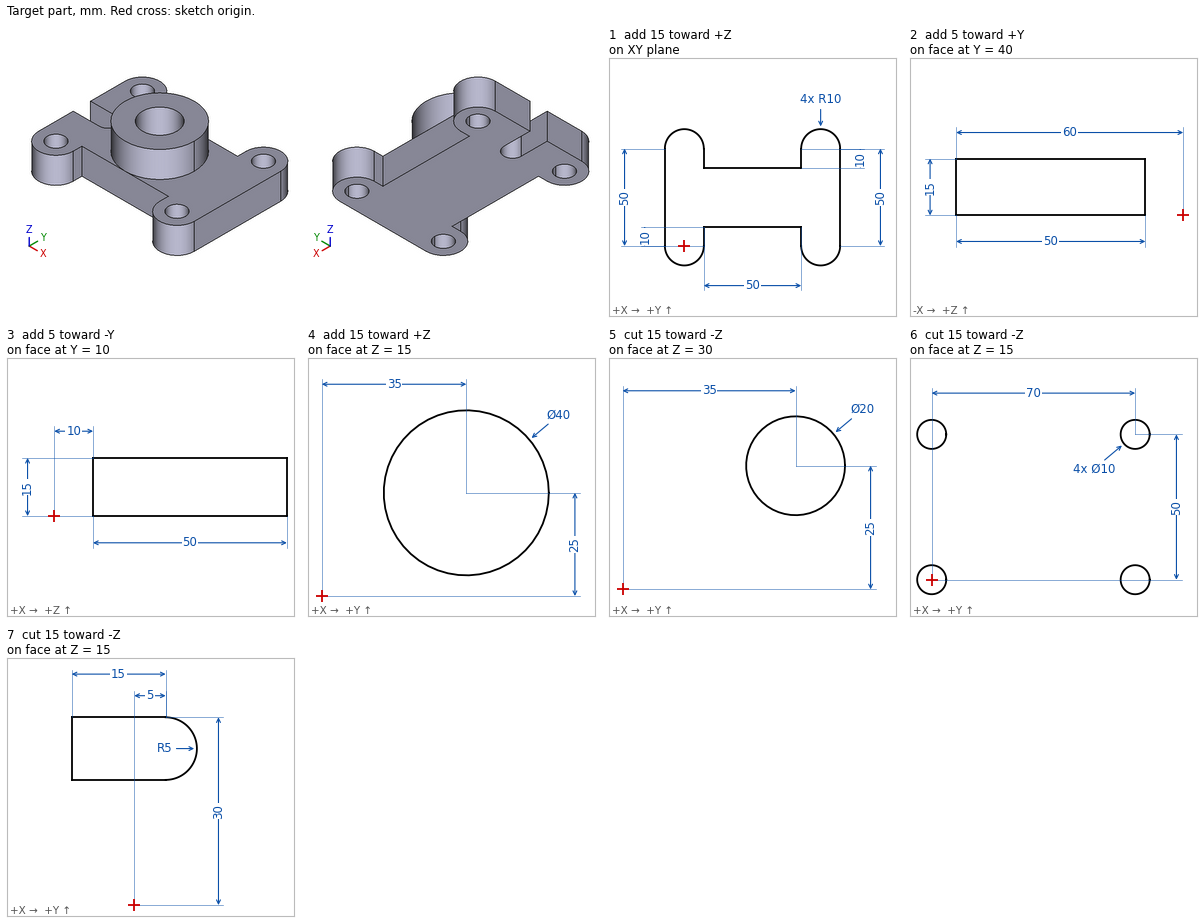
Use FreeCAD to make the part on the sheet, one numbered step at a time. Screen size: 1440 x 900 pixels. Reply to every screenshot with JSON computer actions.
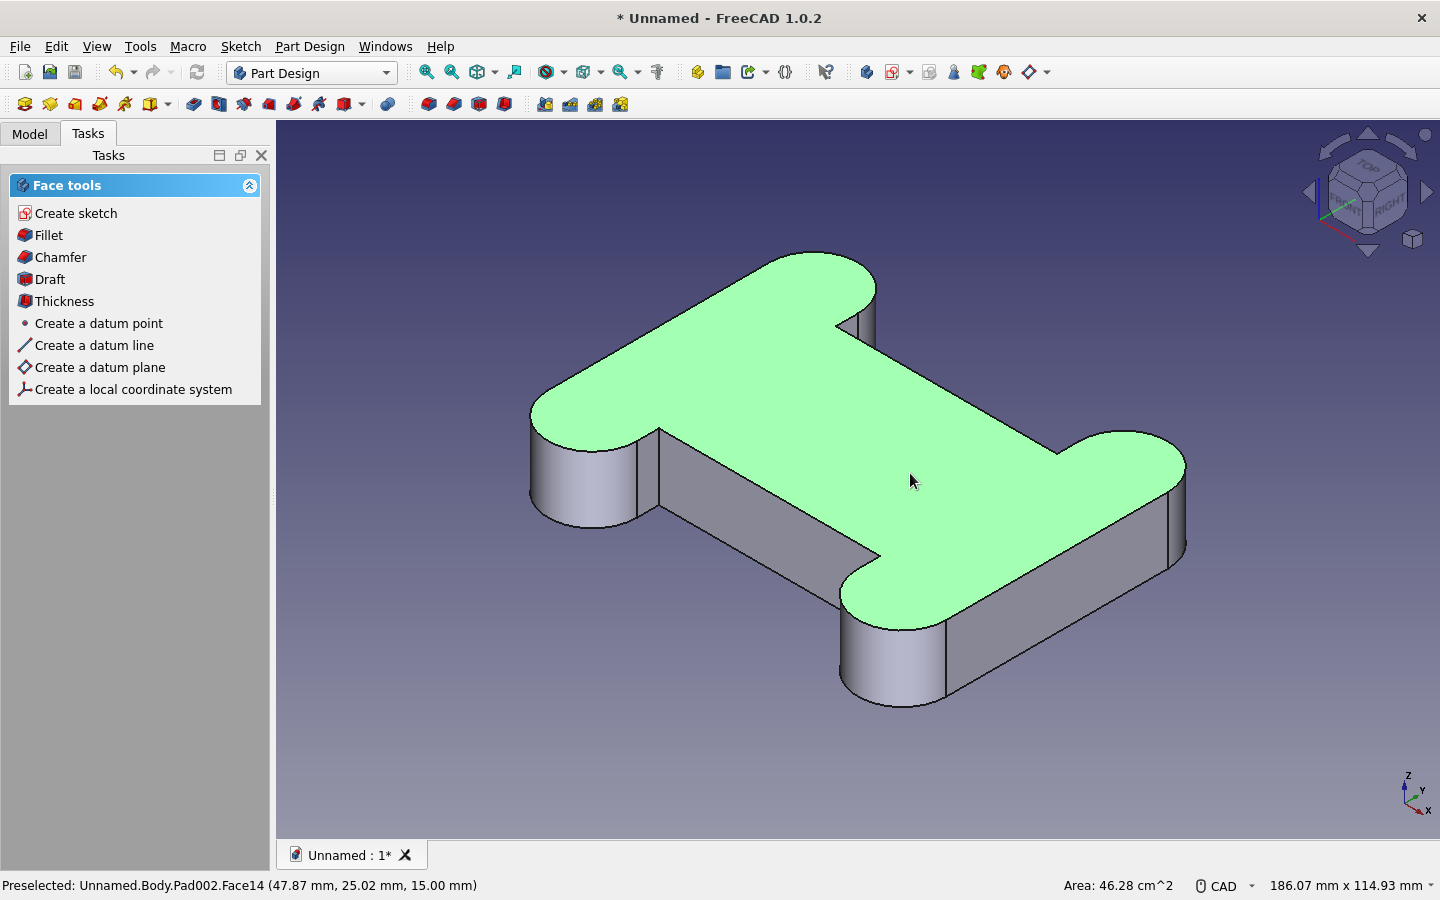
{"action": "left_click", "coordinate": [892, 72]}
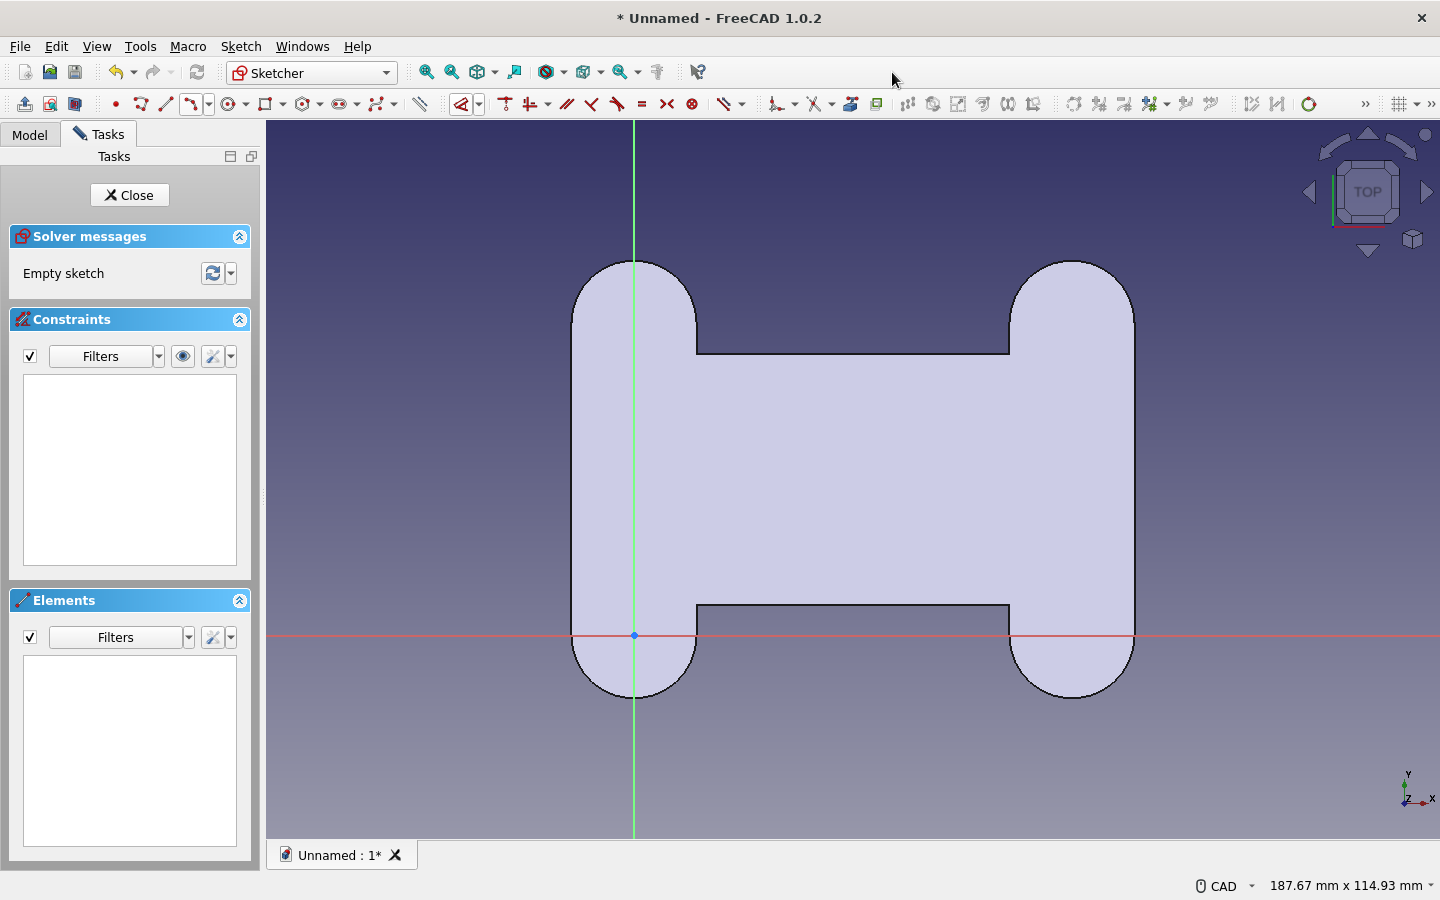
{"action": "scroll", "coordinate": [832, 514], "scroll_direction": "up", "scroll_amount": 3}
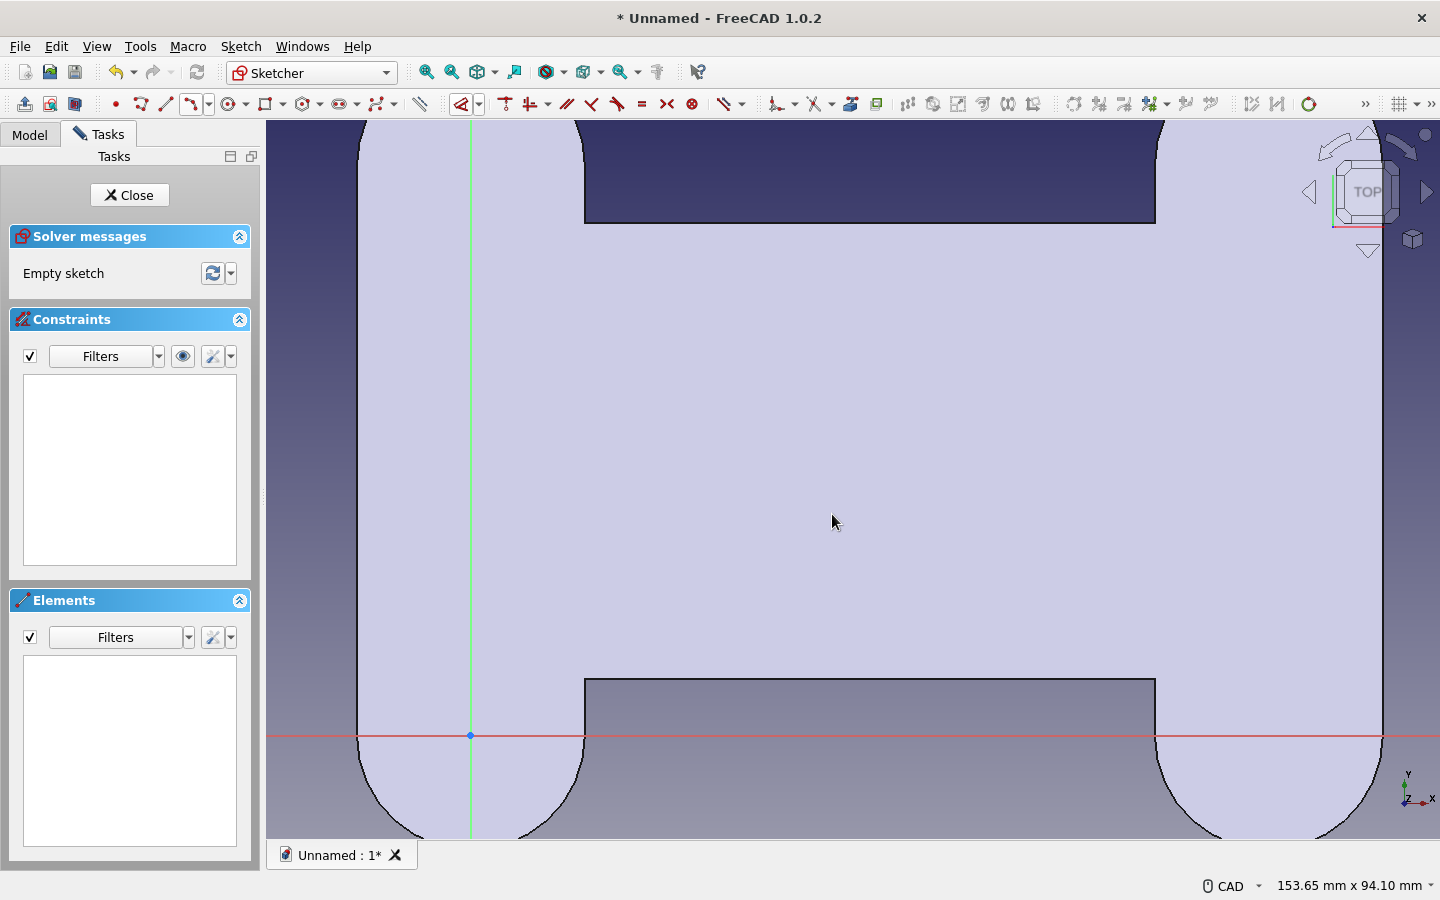
{"action": "left_click", "coordinate": [228, 104]}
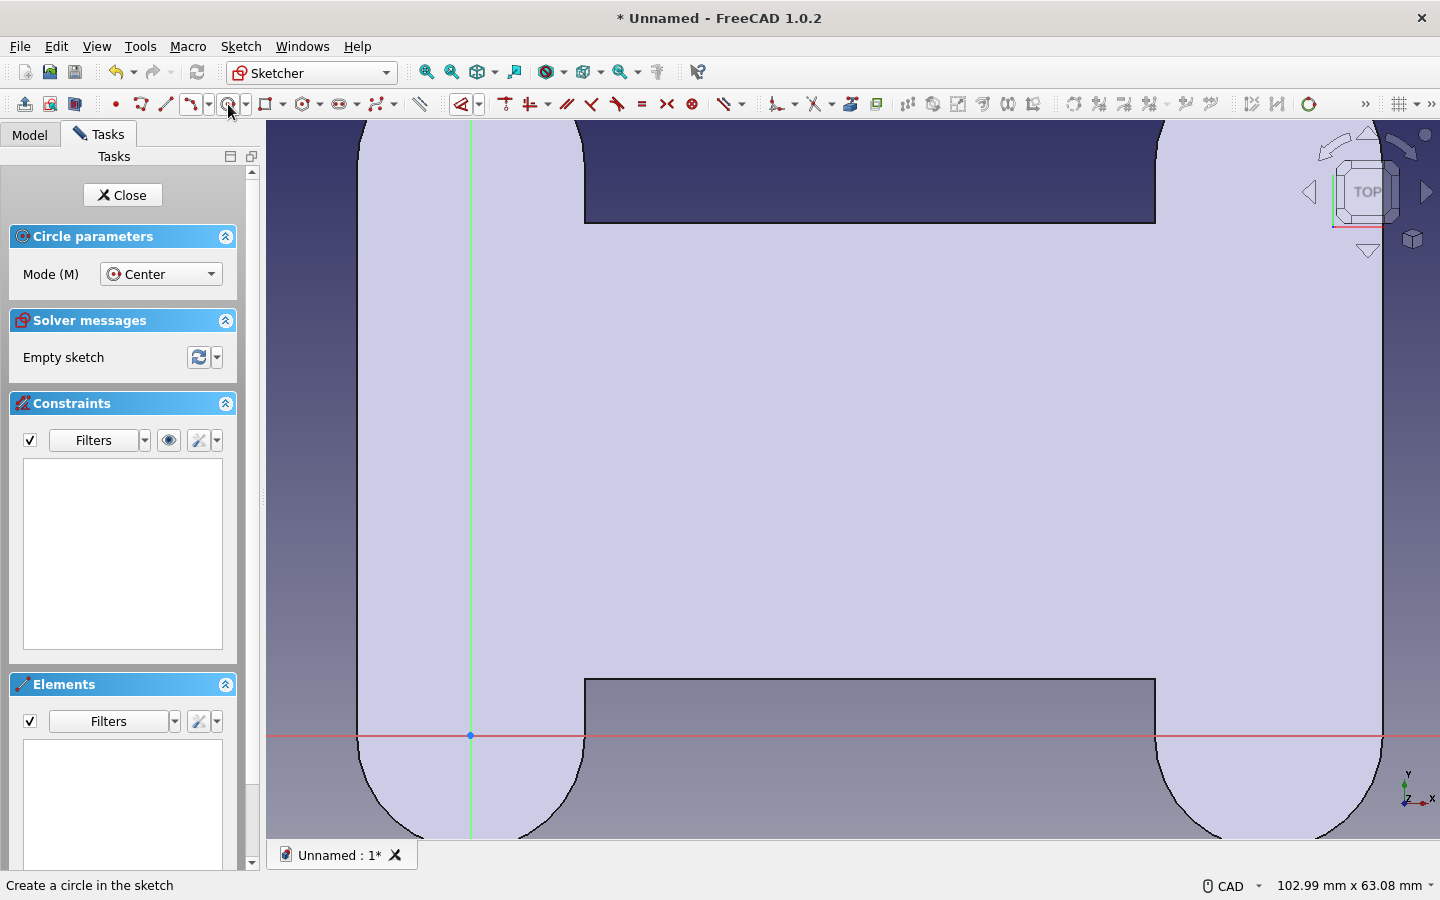
{"action": "left_click", "coordinate": [870, 451]}
{"action": "left_click", "coordinate": [1031, 289]}
{"action": "key", "text": "Escape"}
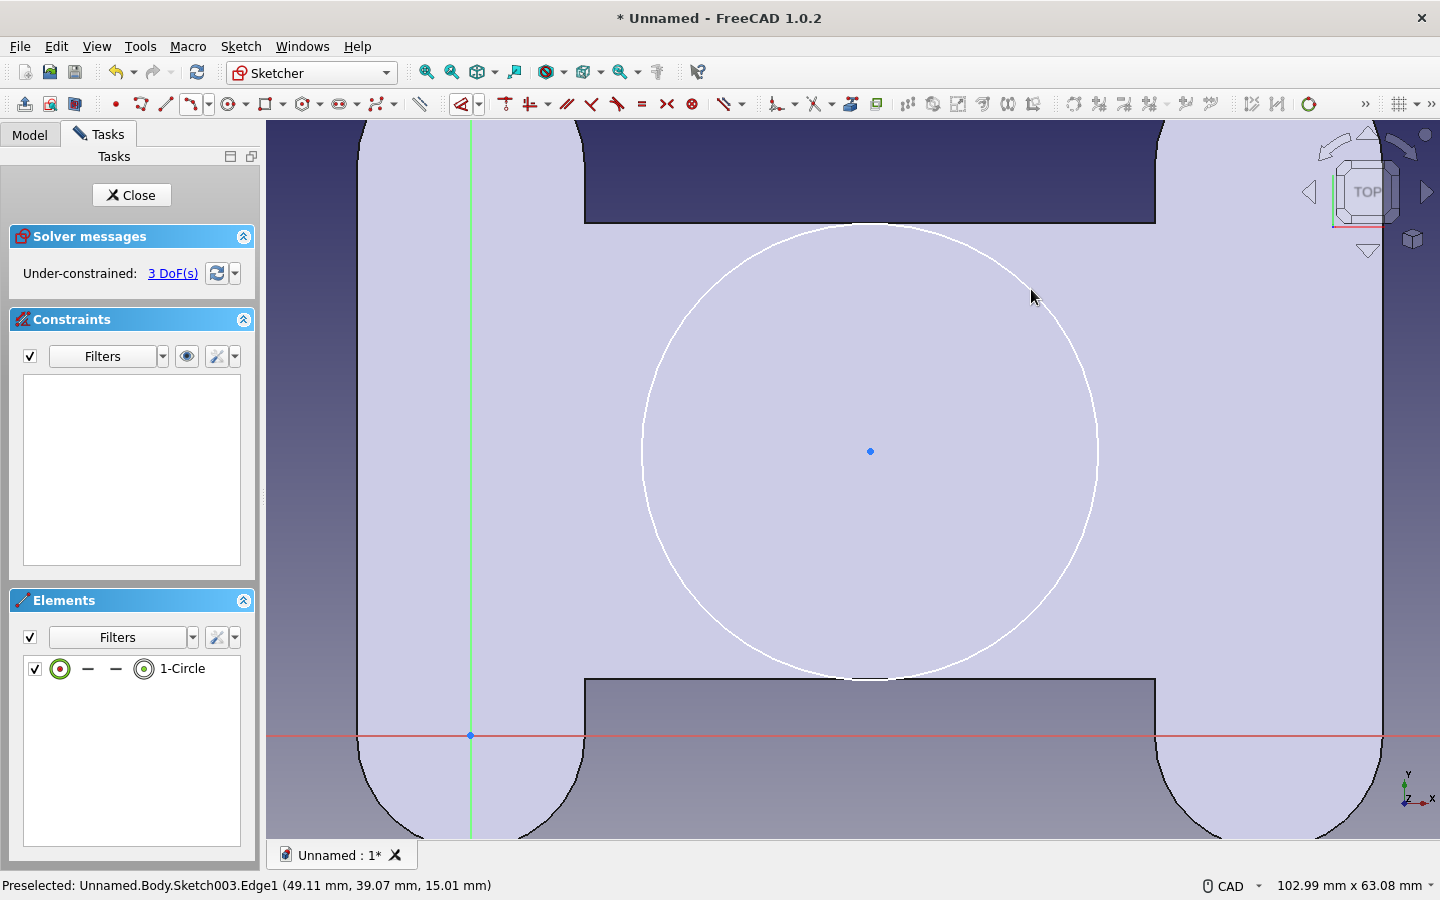
{"action": "left_click", "coordinate": [1031, 290]}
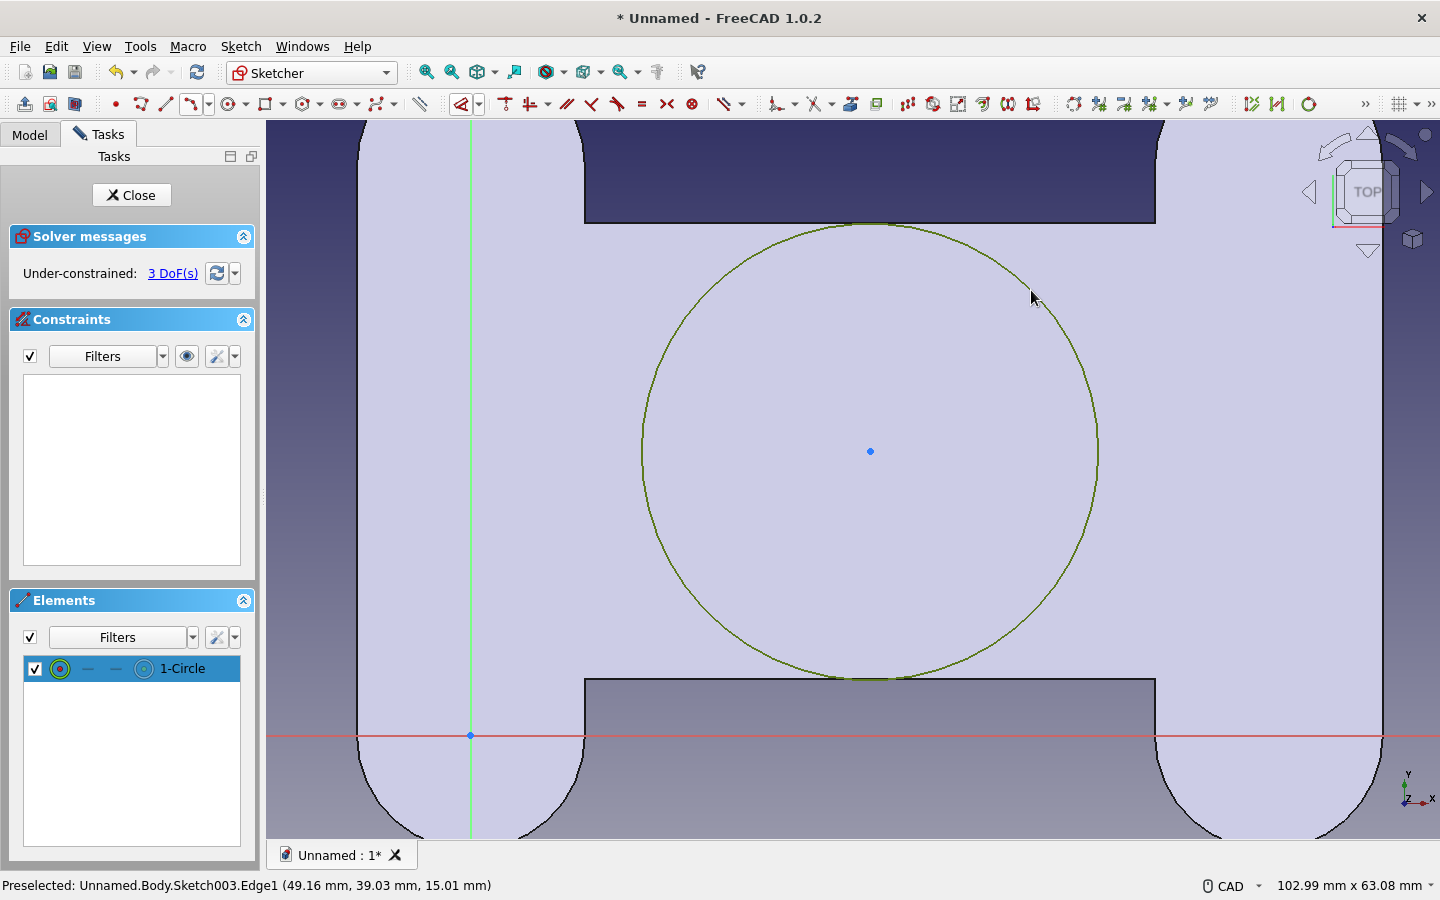
{"action": "left_click", "coordinate": [478, 104]}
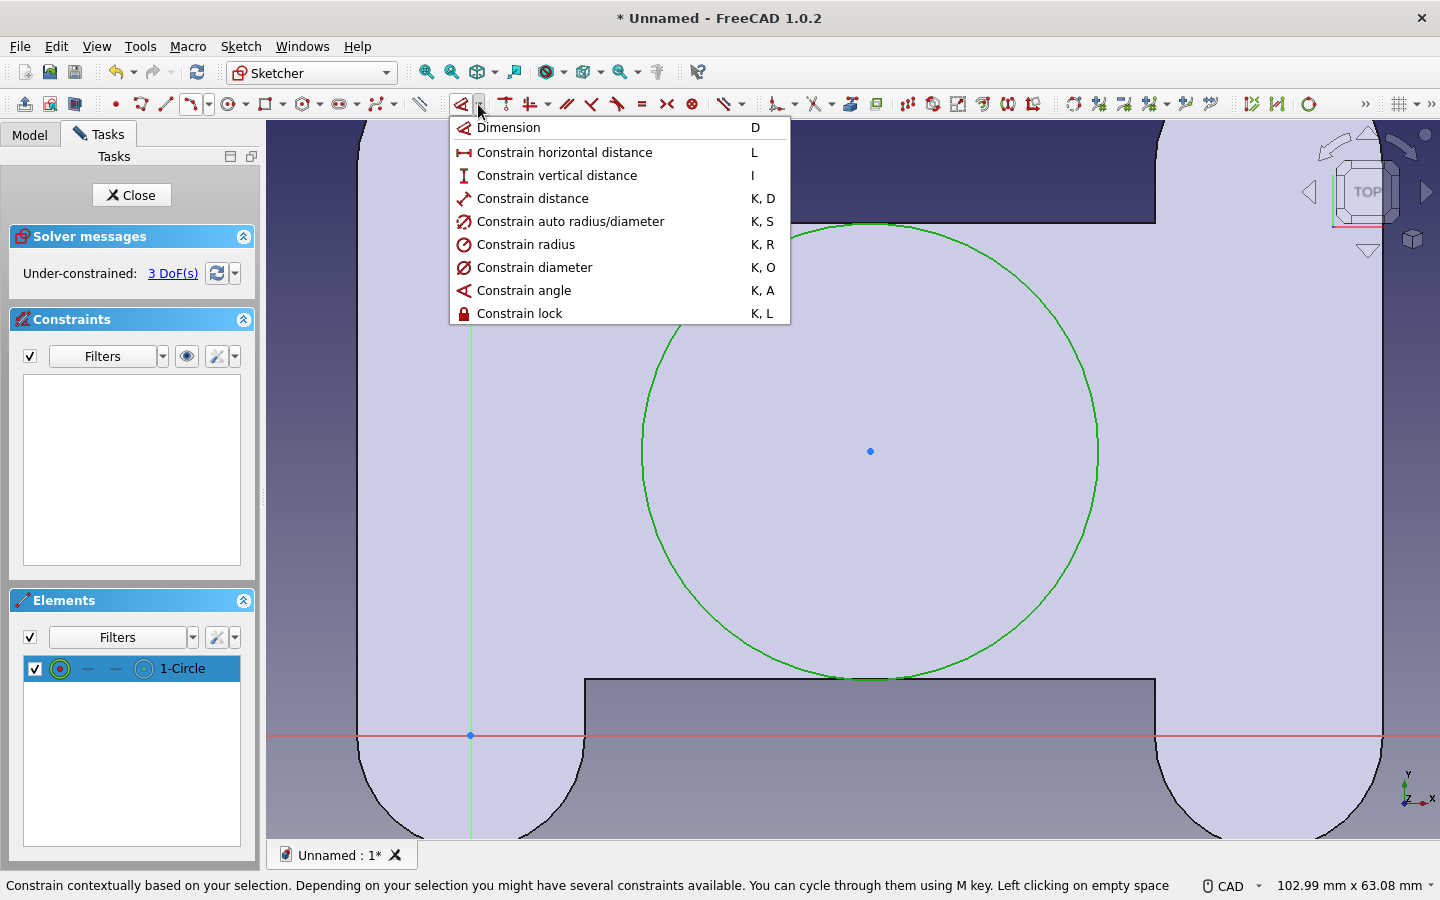
{"action": "left_click", "coordinate": [620, 268]}